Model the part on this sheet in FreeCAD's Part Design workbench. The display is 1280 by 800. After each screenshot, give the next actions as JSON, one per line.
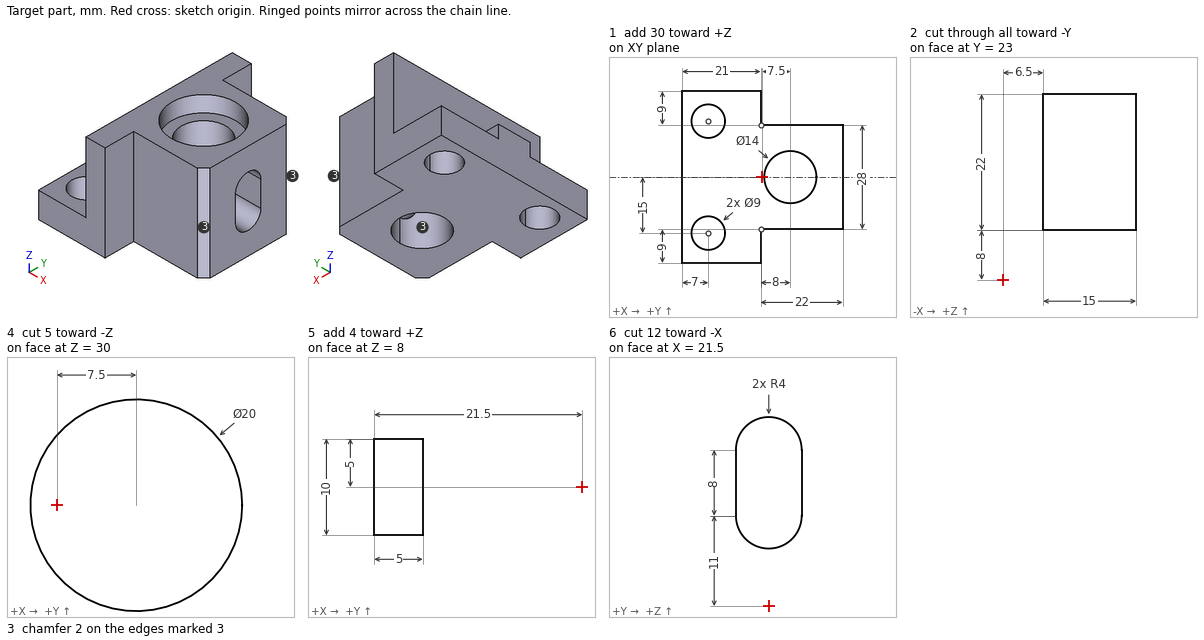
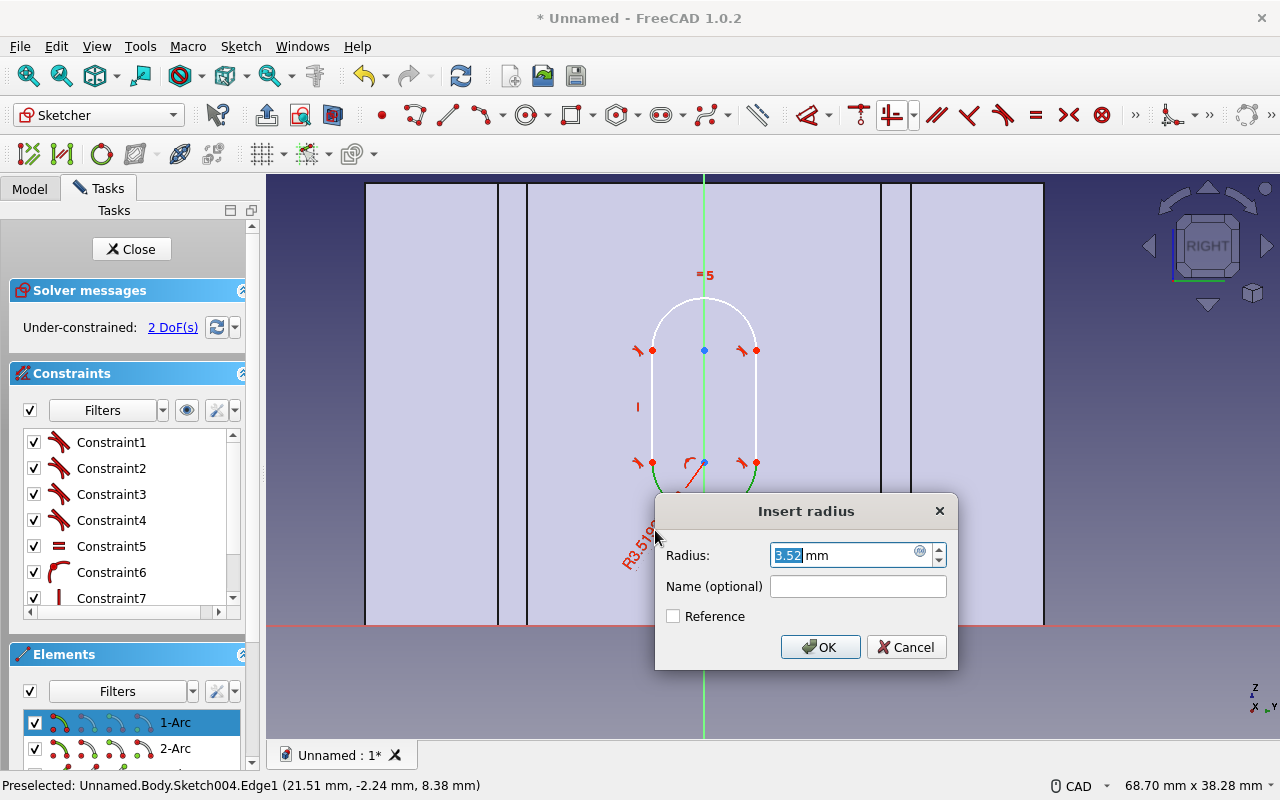
{"action": "type", "text": "4"}
{"action": "key", "text": "Return"}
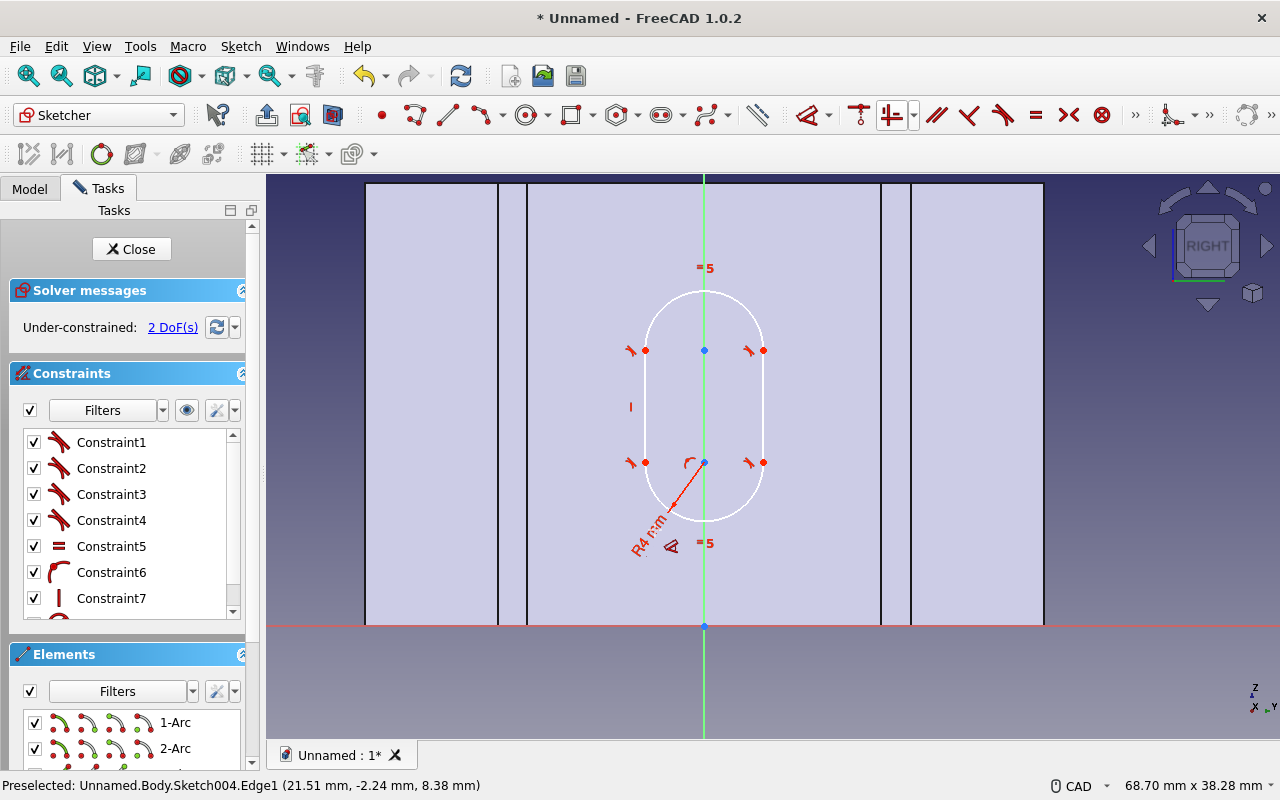
{"action": "left_click", "coordinate": [645, 429]}
{"action": "left_click", "coordinate": [611, 406]}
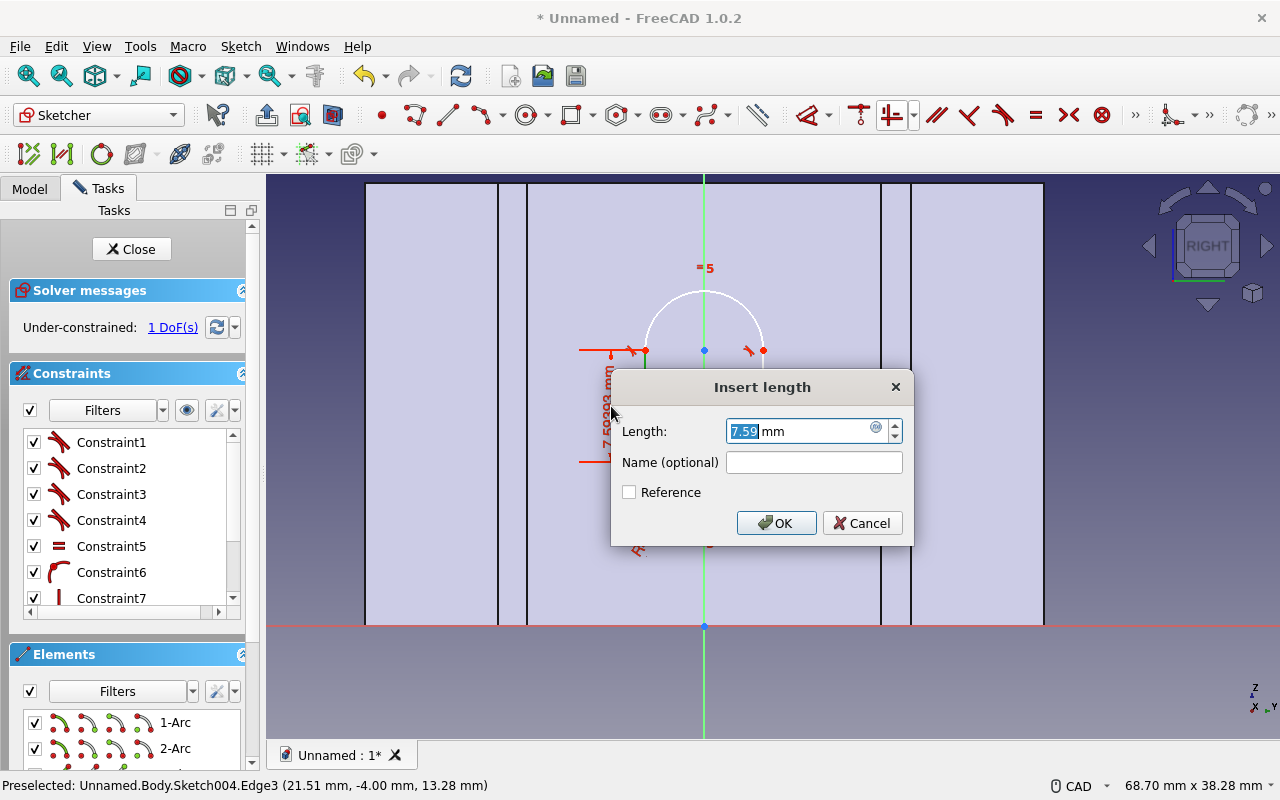
{"action": "type", "text": "8"}
{"action": "key", "text": "Return"}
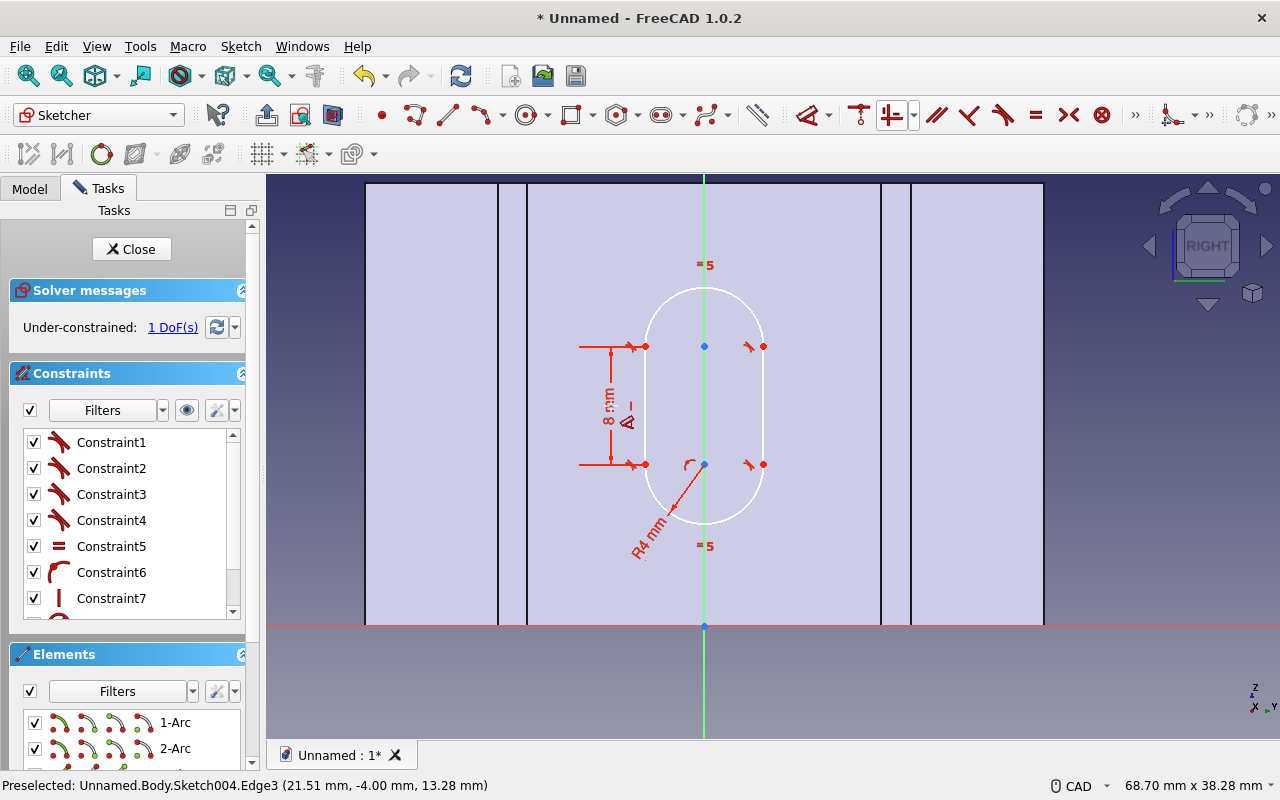
{"action": "left_click", "coordinate": [645, 465]}
{"action": "left_click", "coordinate": [611, 508]}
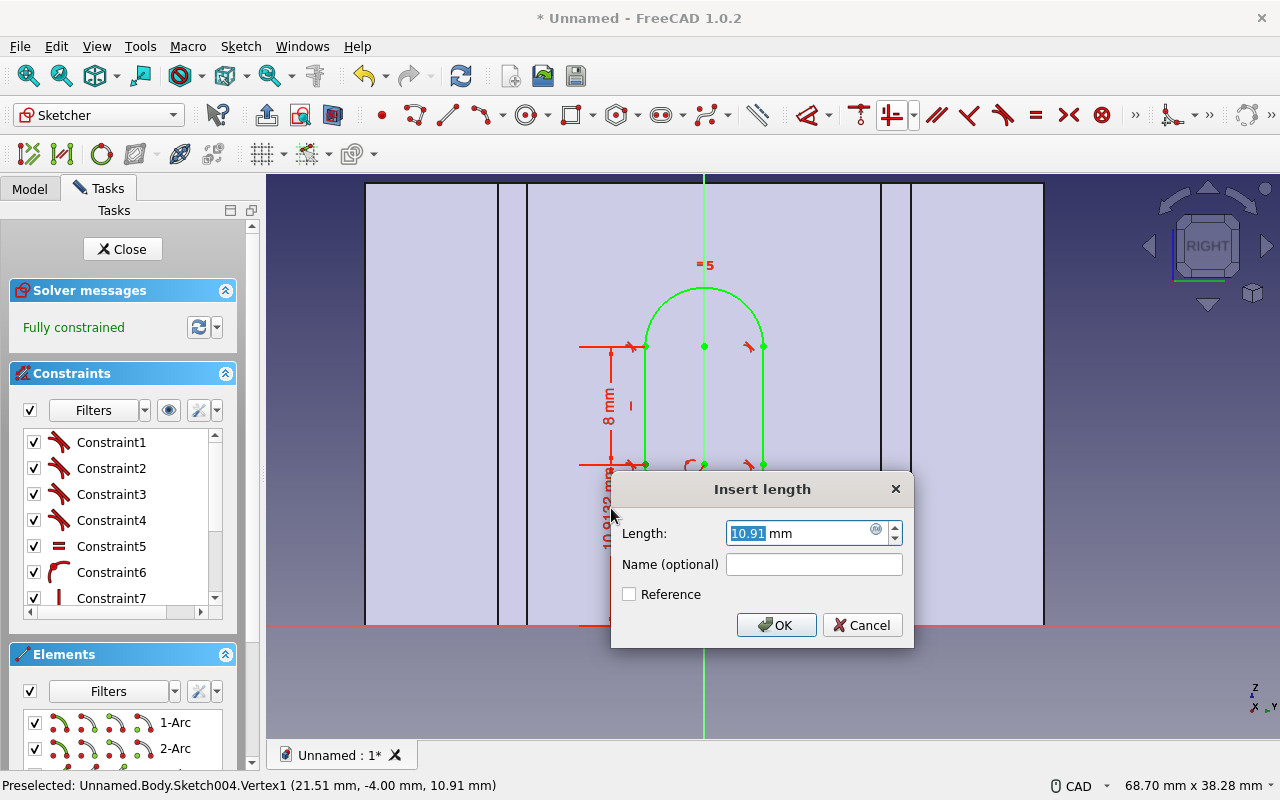
{"action": "type", "text": "11"}
{"action": "key", "text": "Return"}
{"action": "key", "text": "Escape"}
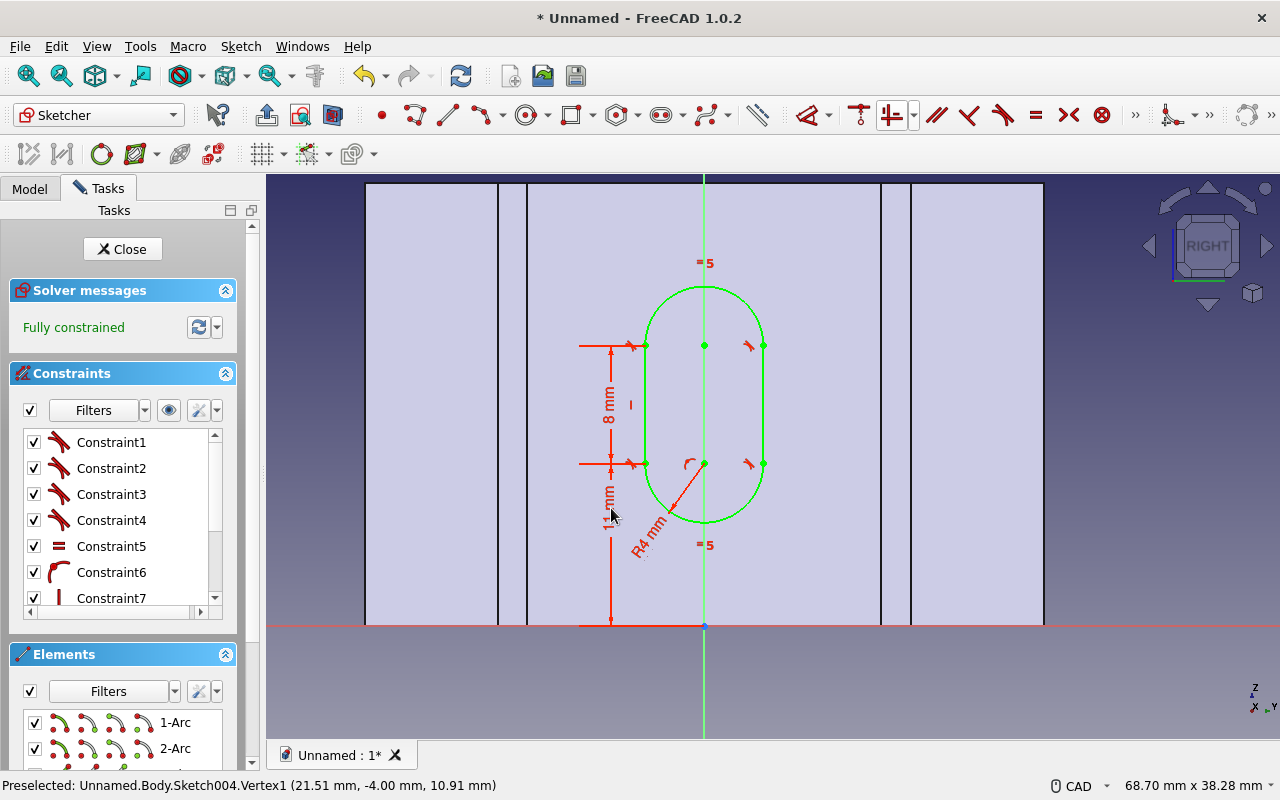
{"action": "left_click", "coordinate": [123, 249]}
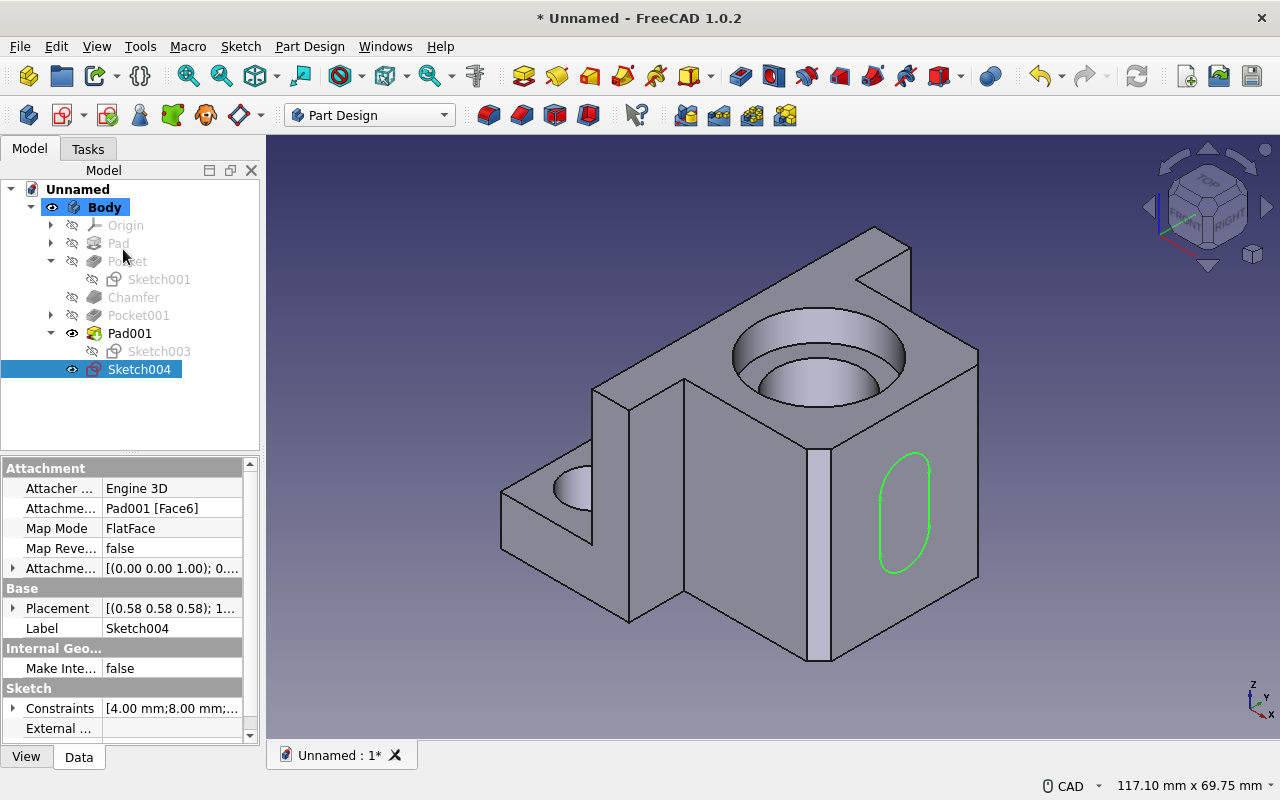
{"action": "left_click", "coordinate": [741, 76]}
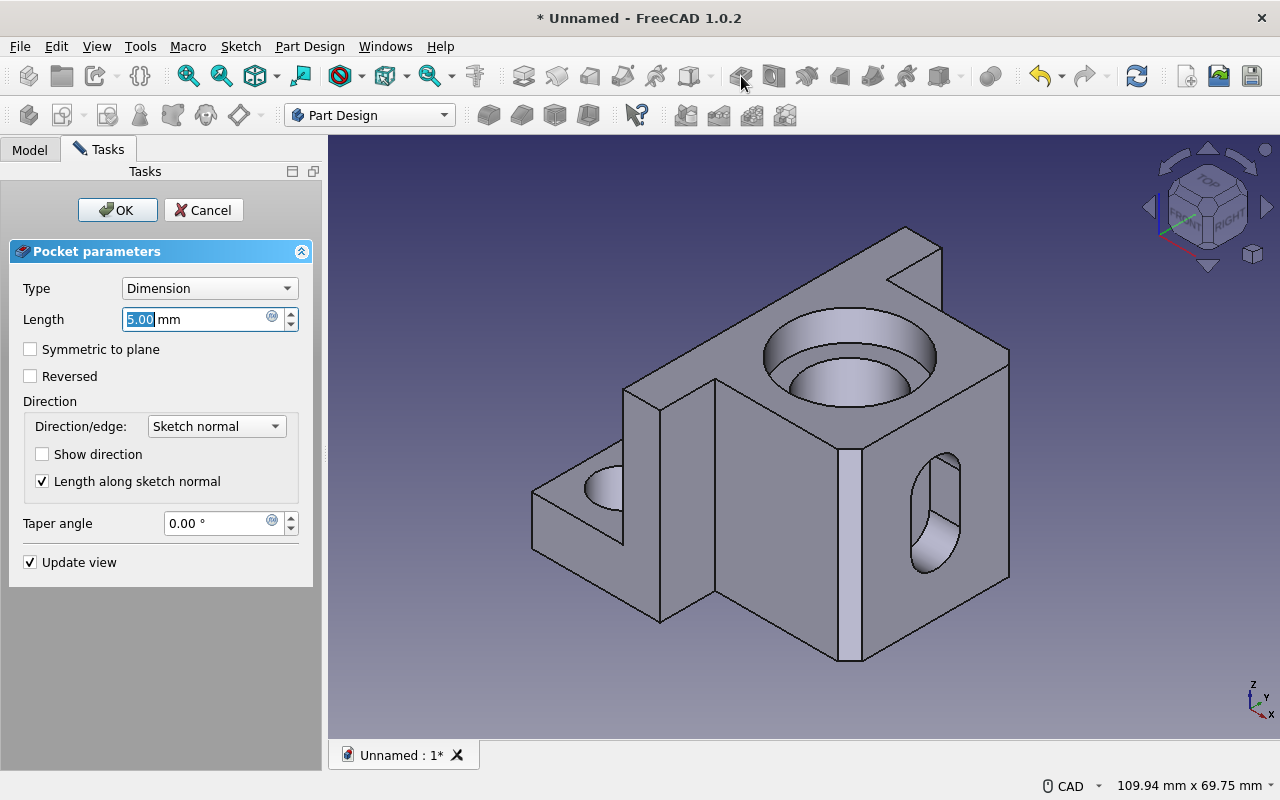
{"action": "type", "text": "12"}
{"action": "key", "text": "Tab"}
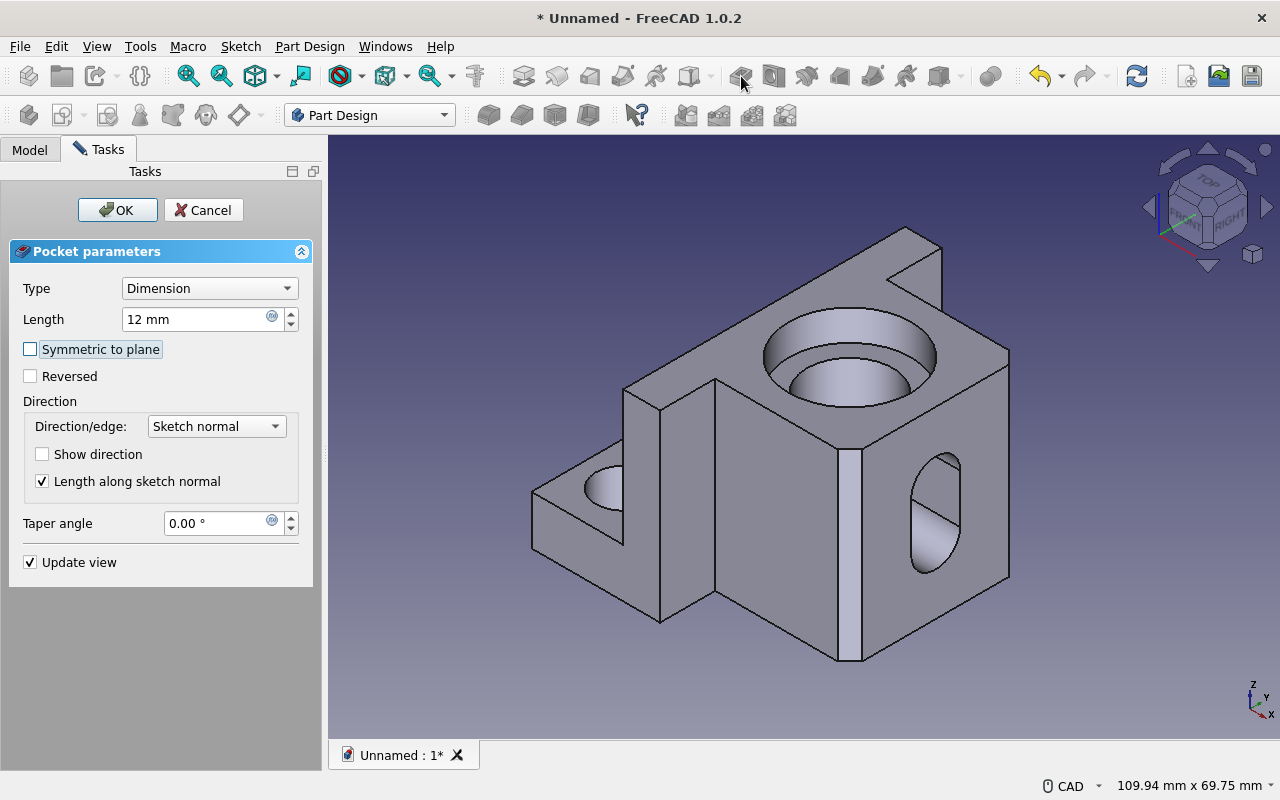
{"action": "left_click", "coordinate": [118, 210]}